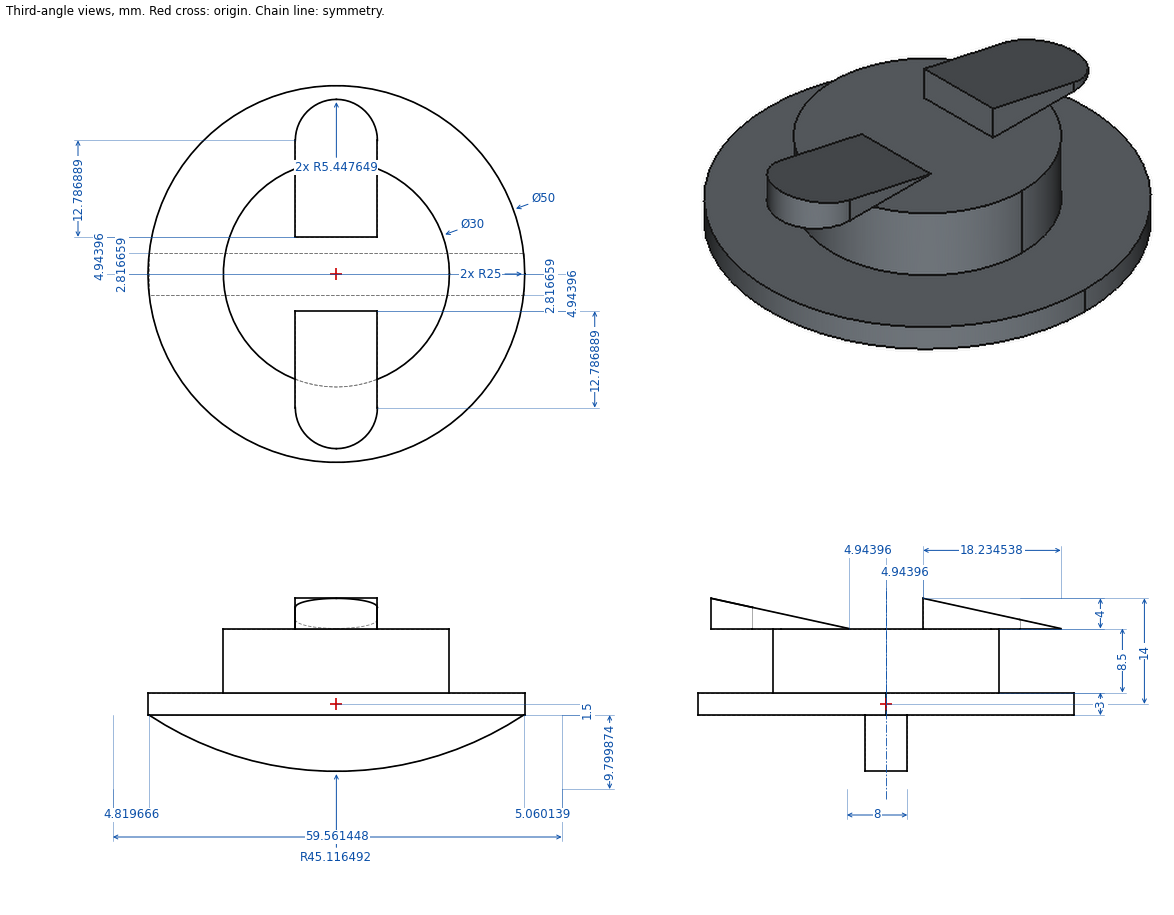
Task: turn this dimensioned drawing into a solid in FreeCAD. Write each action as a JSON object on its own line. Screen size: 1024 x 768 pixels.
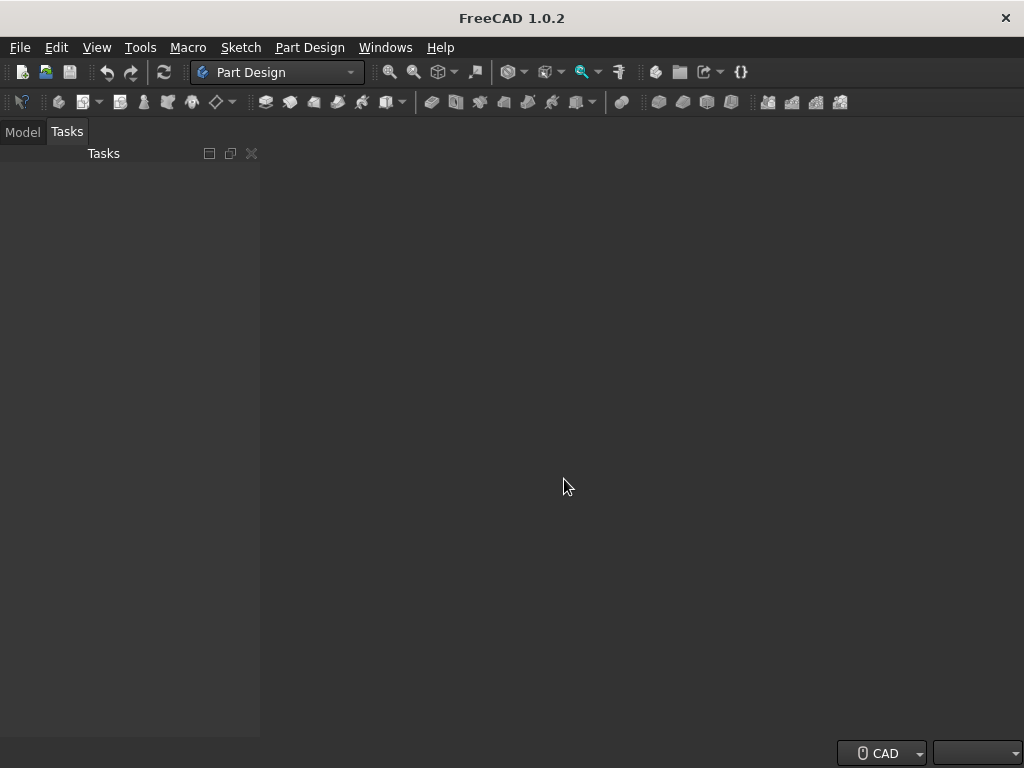
{"action": "left_click", "coordinate": [22, 72]}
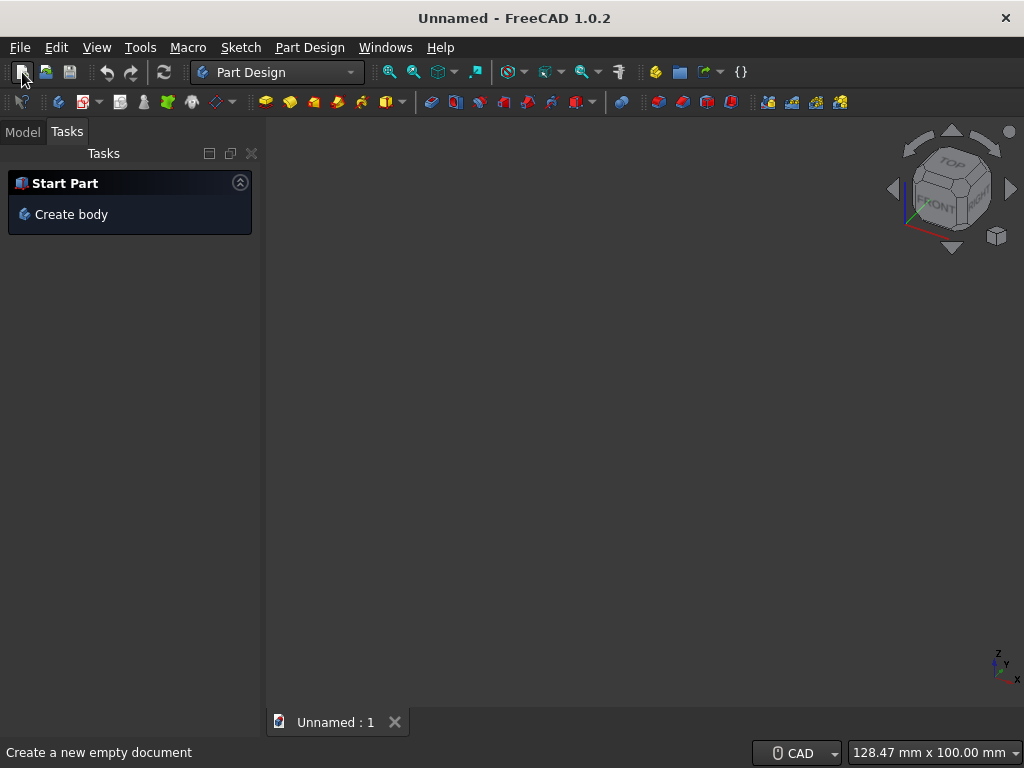
{"action": "left_click", "coordinate": [84, 102]}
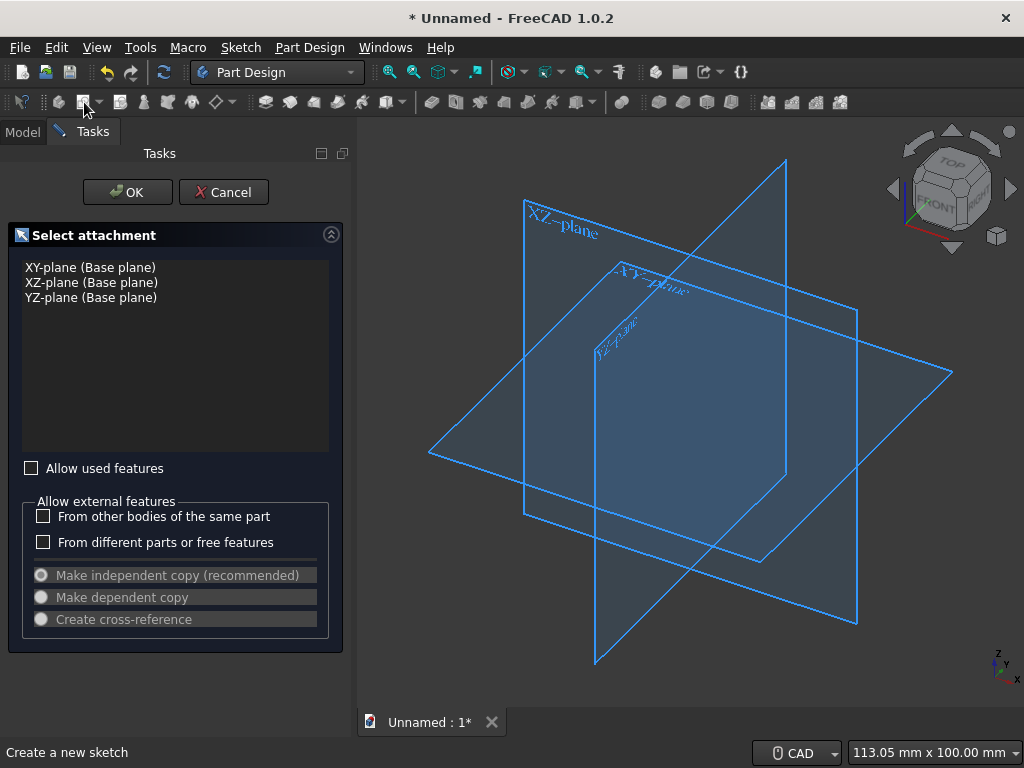
{"action": "left_click", "coordinate": [82, 268]}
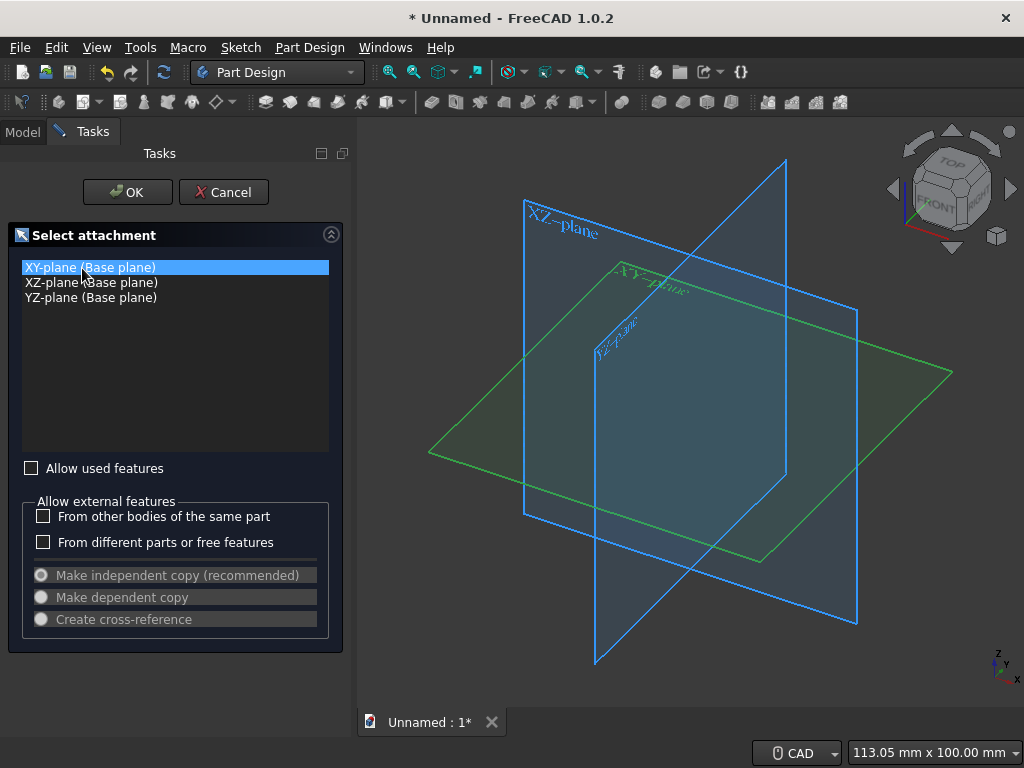
{"action": "left_click", "coordinate": [128, 192]}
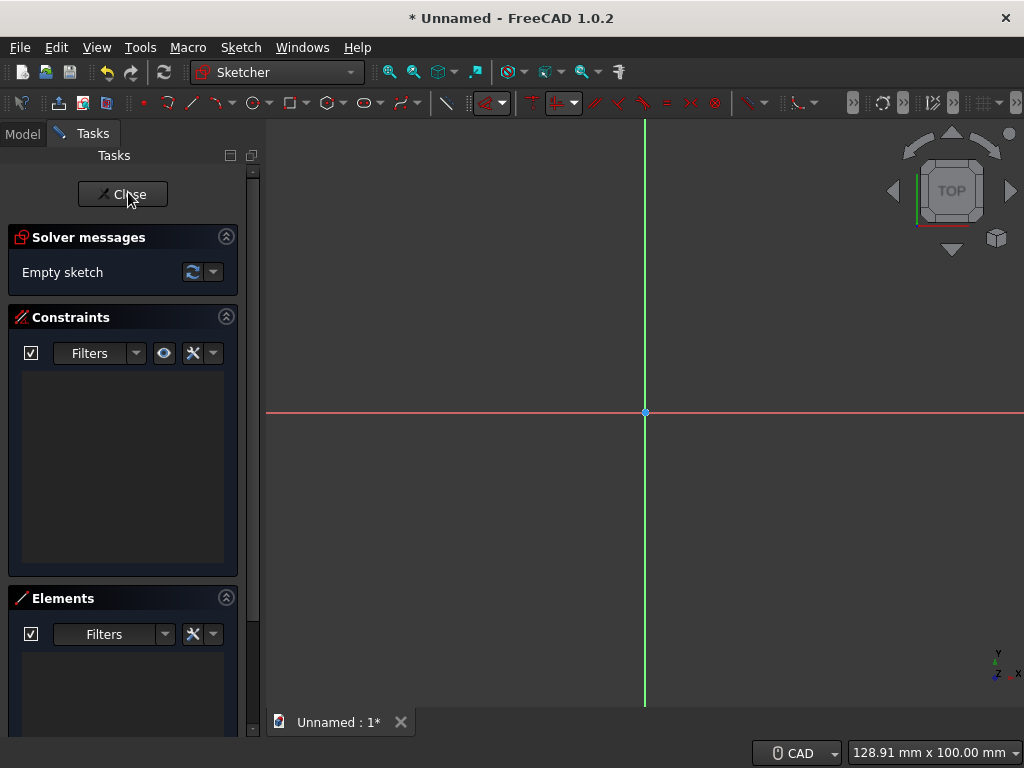
{"action": "left_click", "coordinate": [254, 104]}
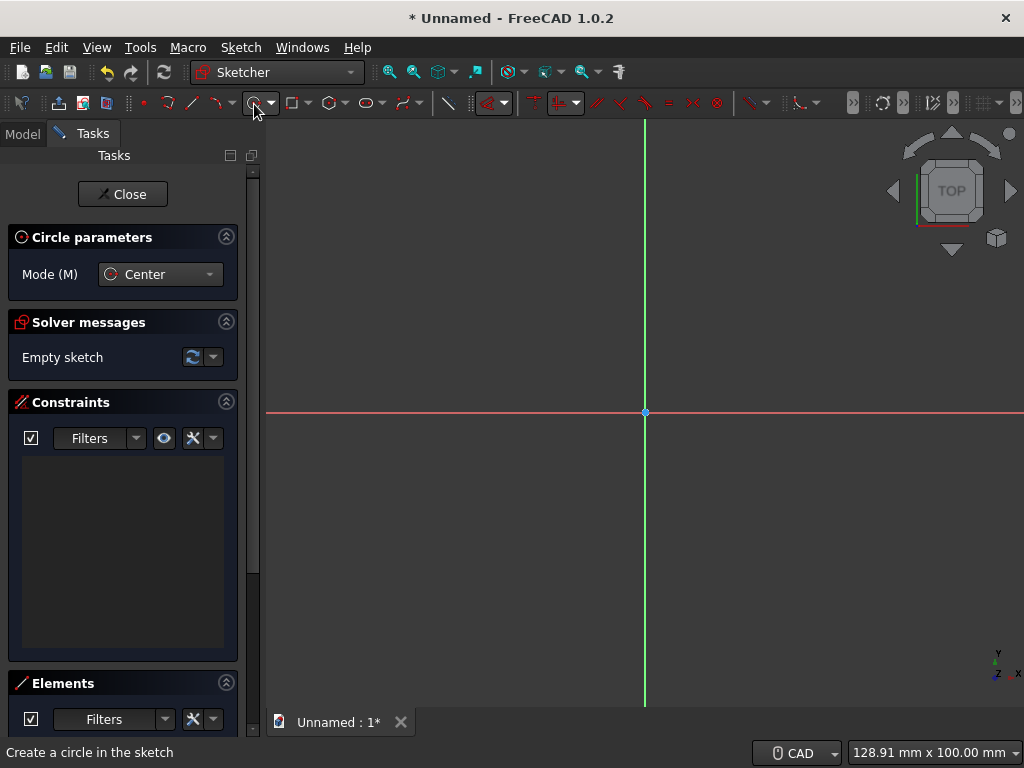
{"action": "left_click", "coordinate": [645, 413]}
{"action": "left_click", "coordinate": [749, 309]}
{"action": "key", "text": "Escape"}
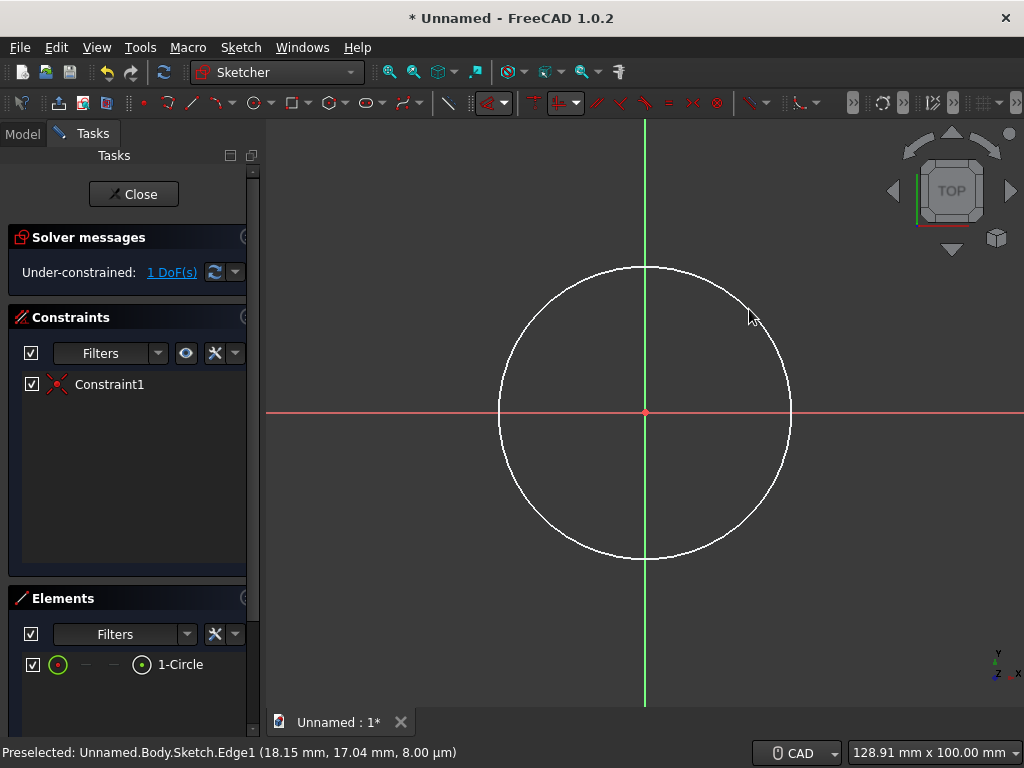
{"action": "left_click", "coordinate": [488, 104]}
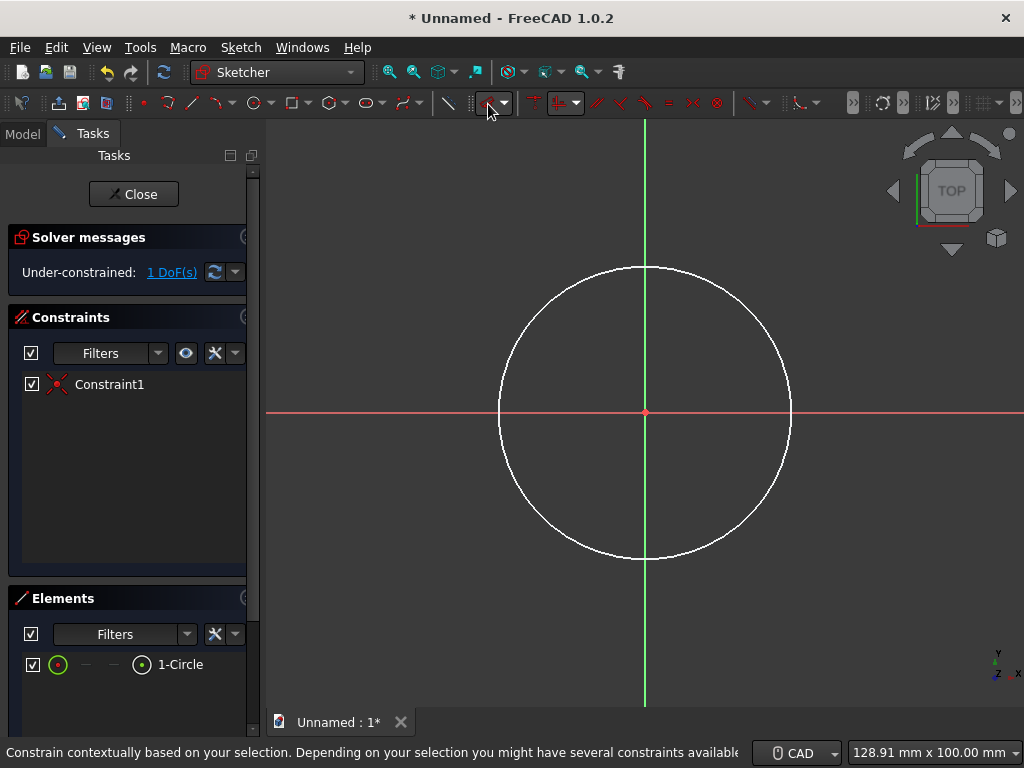
{"action": "left_click", "coordinate": [748, 309]}
{"action": "left_click", "coordinate": [771, 286]}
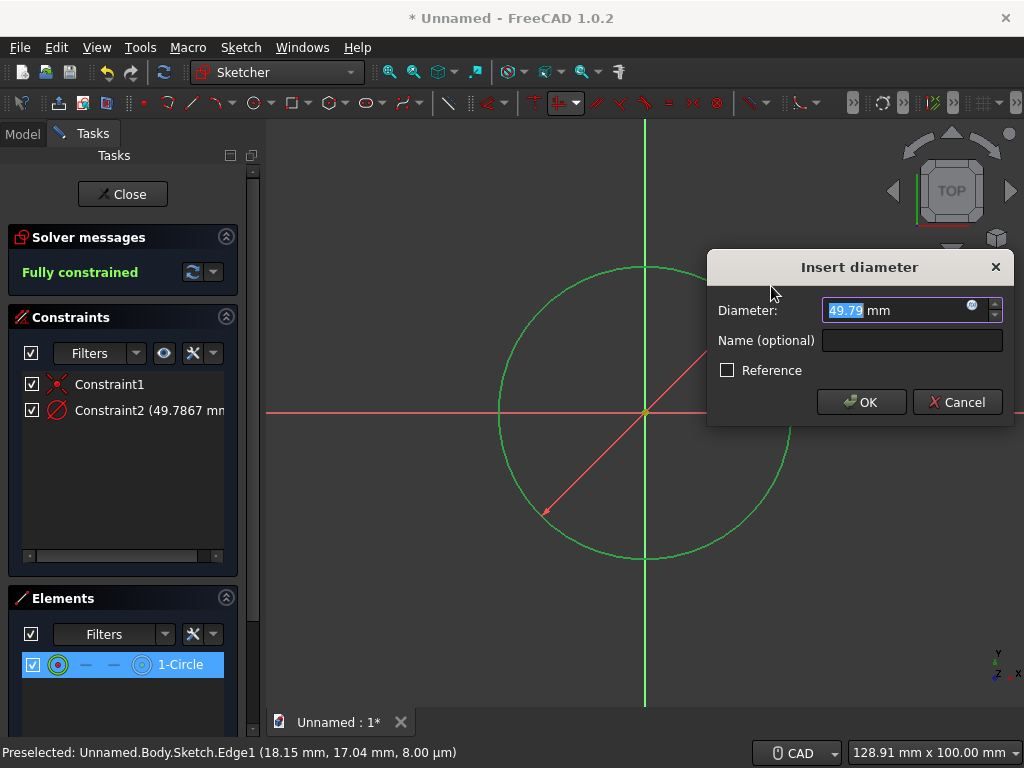
{"action": "type", "text": "50"}
{"action": "key", "text": "Return"}
{"action": "key", "text": "Escape"}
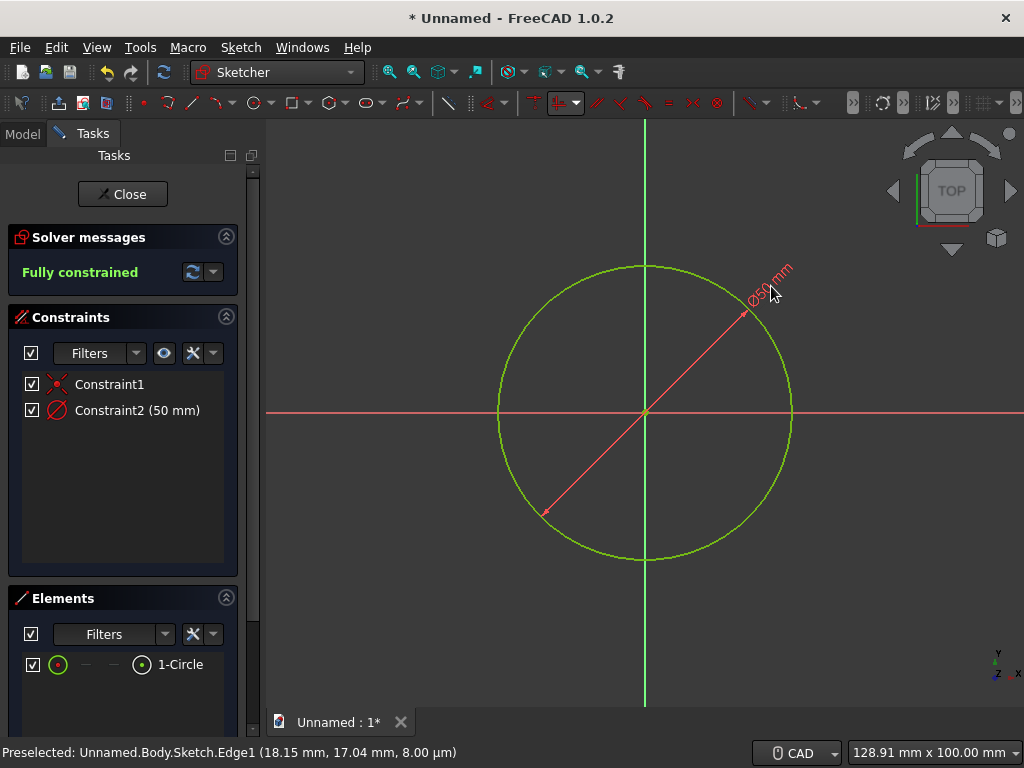
{"action": "left_click", "coordinate": [123, 194]}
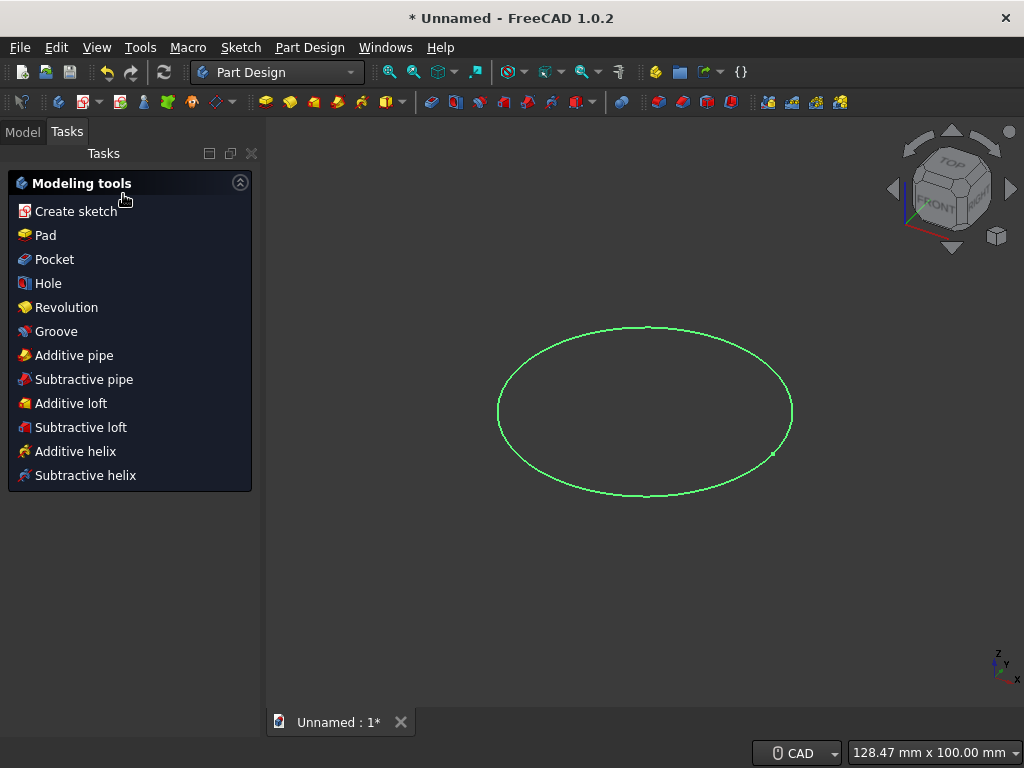
{"action": "left_click", "coordinate": [266, 102]}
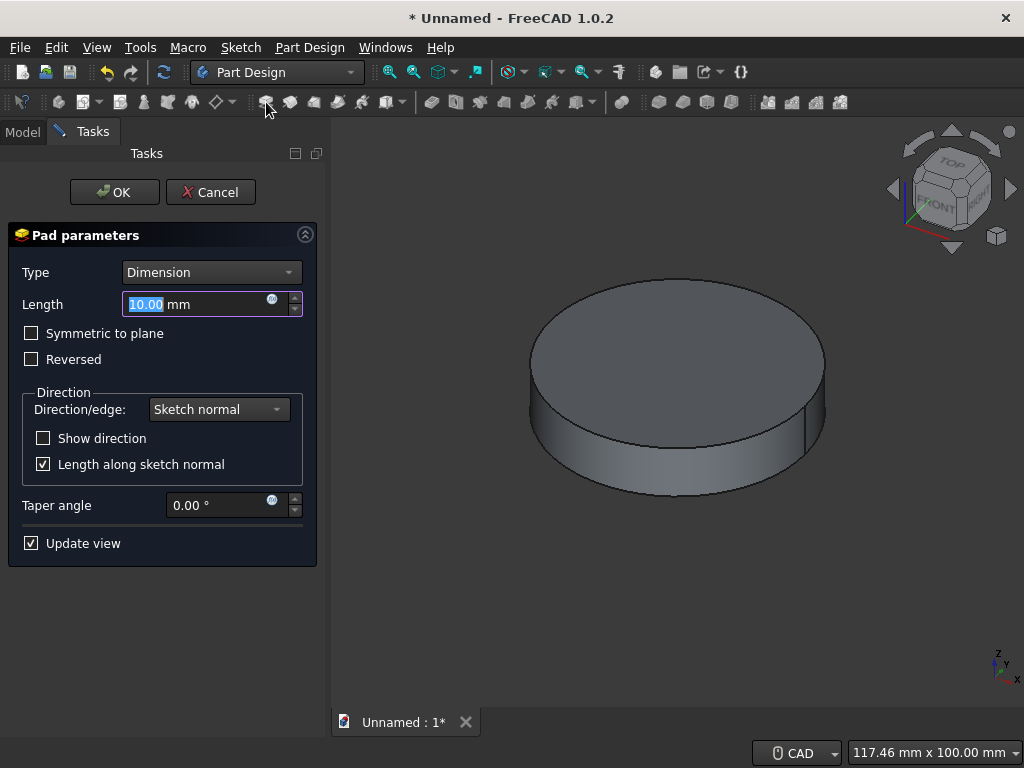
{"action": "type", "text": "3"}
{"action": "key", "text": "Tab"}